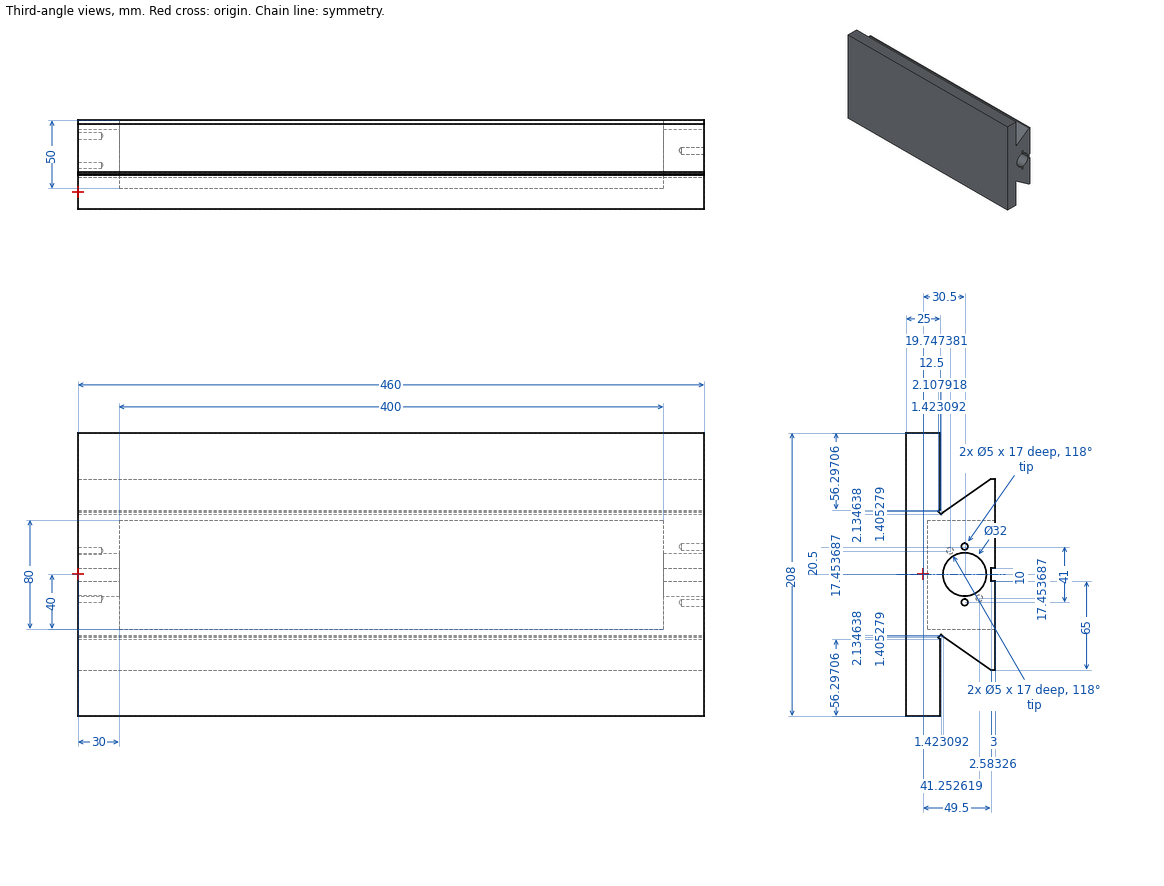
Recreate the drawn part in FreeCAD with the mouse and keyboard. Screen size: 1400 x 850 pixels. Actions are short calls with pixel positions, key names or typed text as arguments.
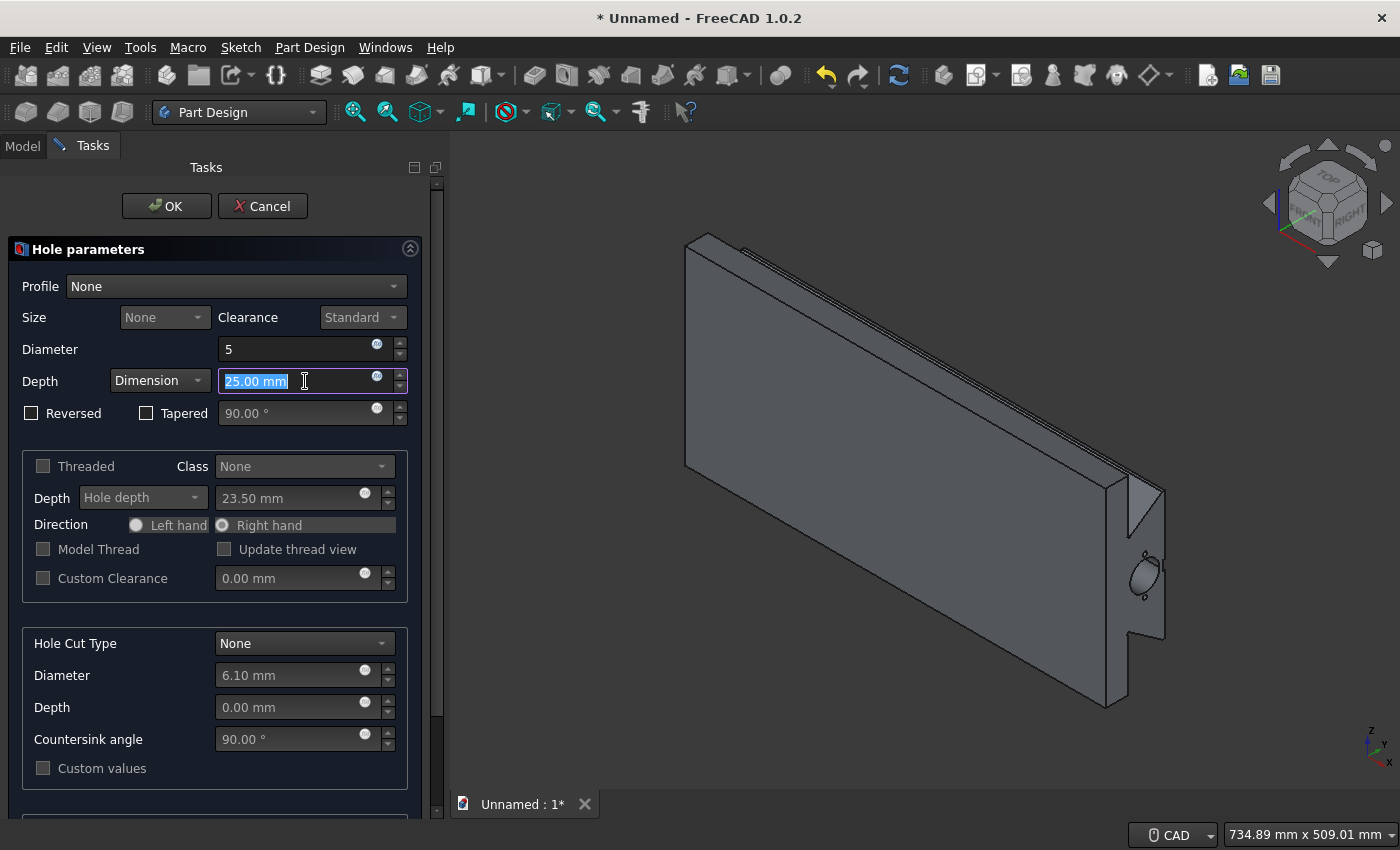
text(17)
key(Tab)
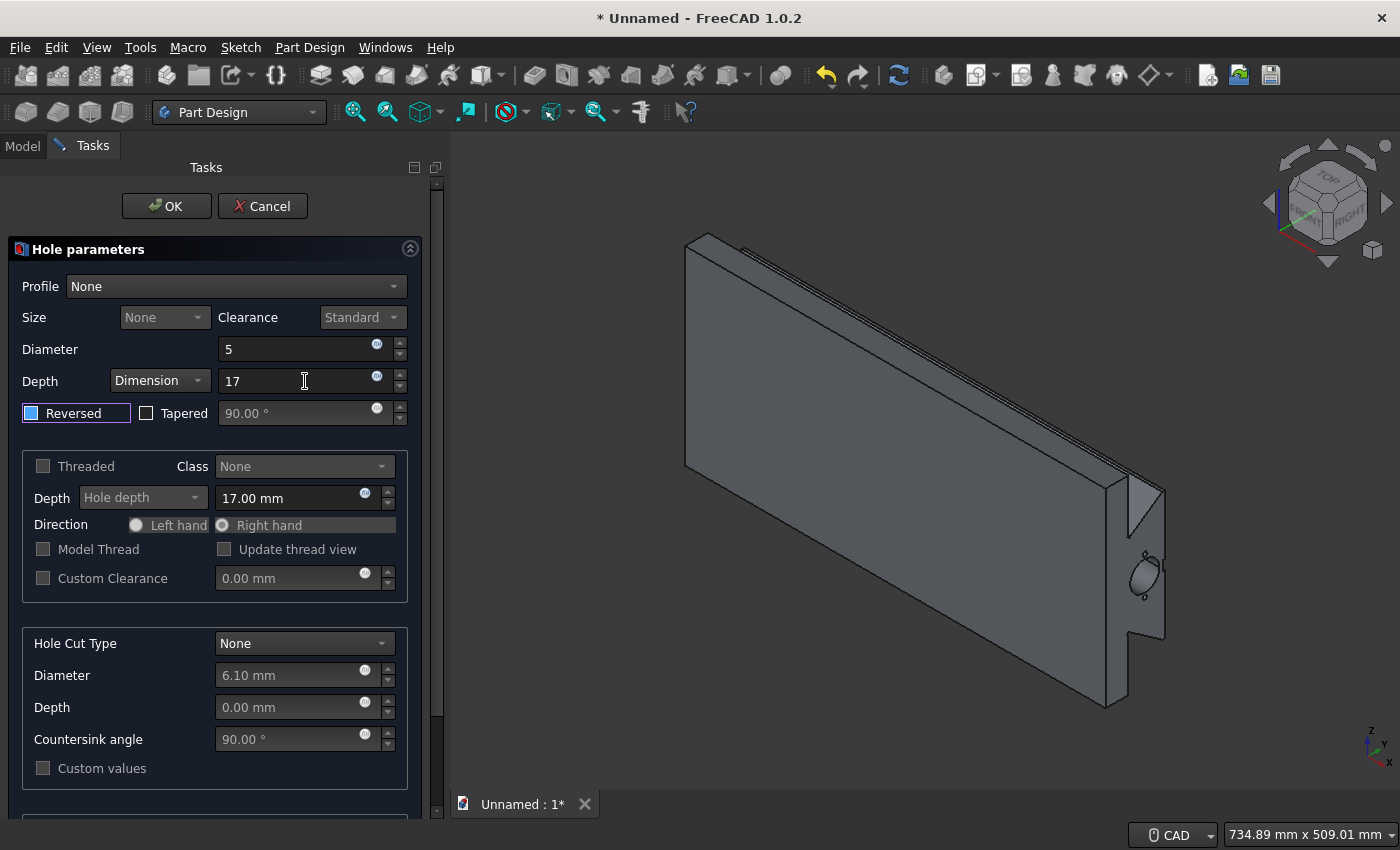
click(167, 206)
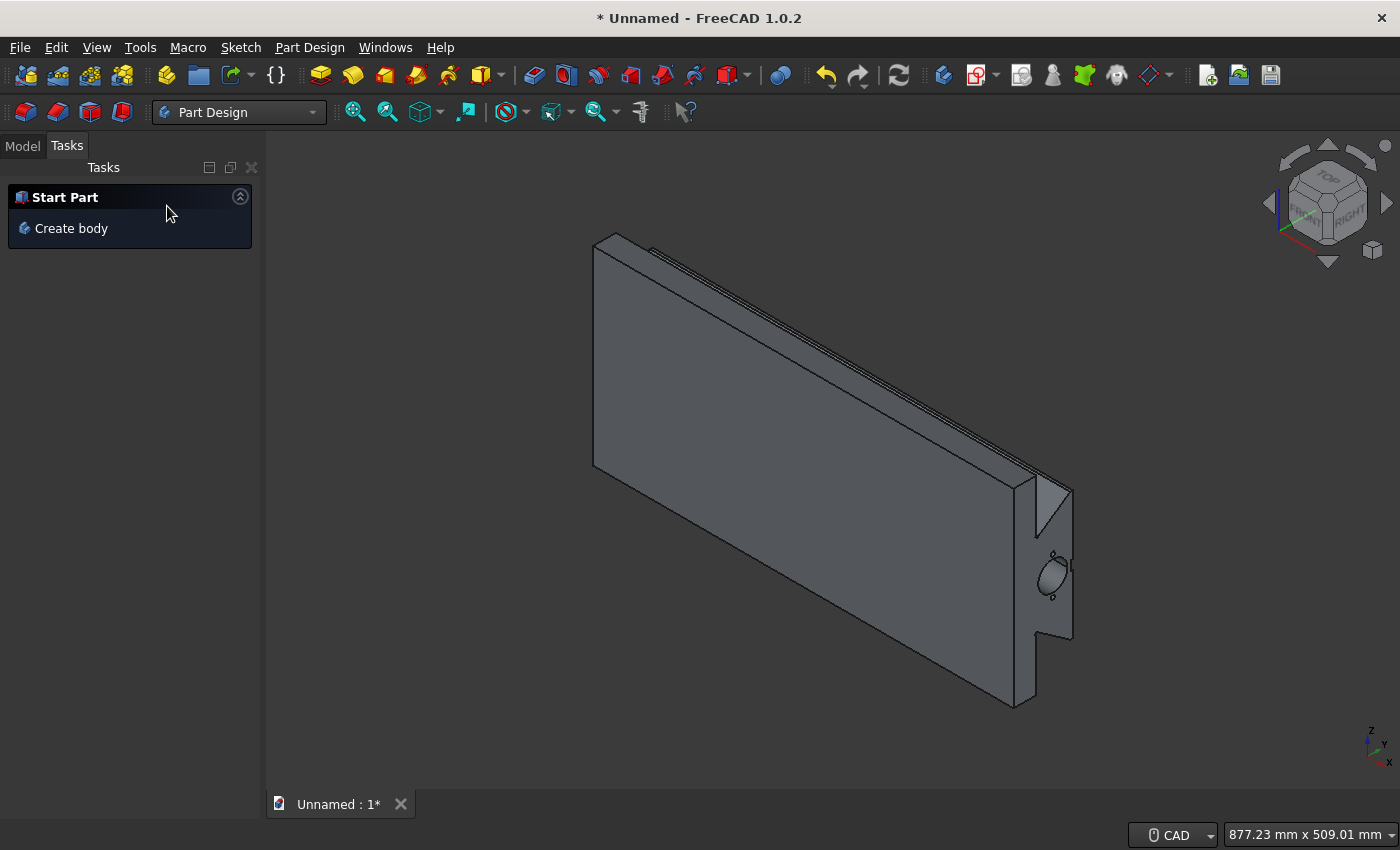
click(976, 76)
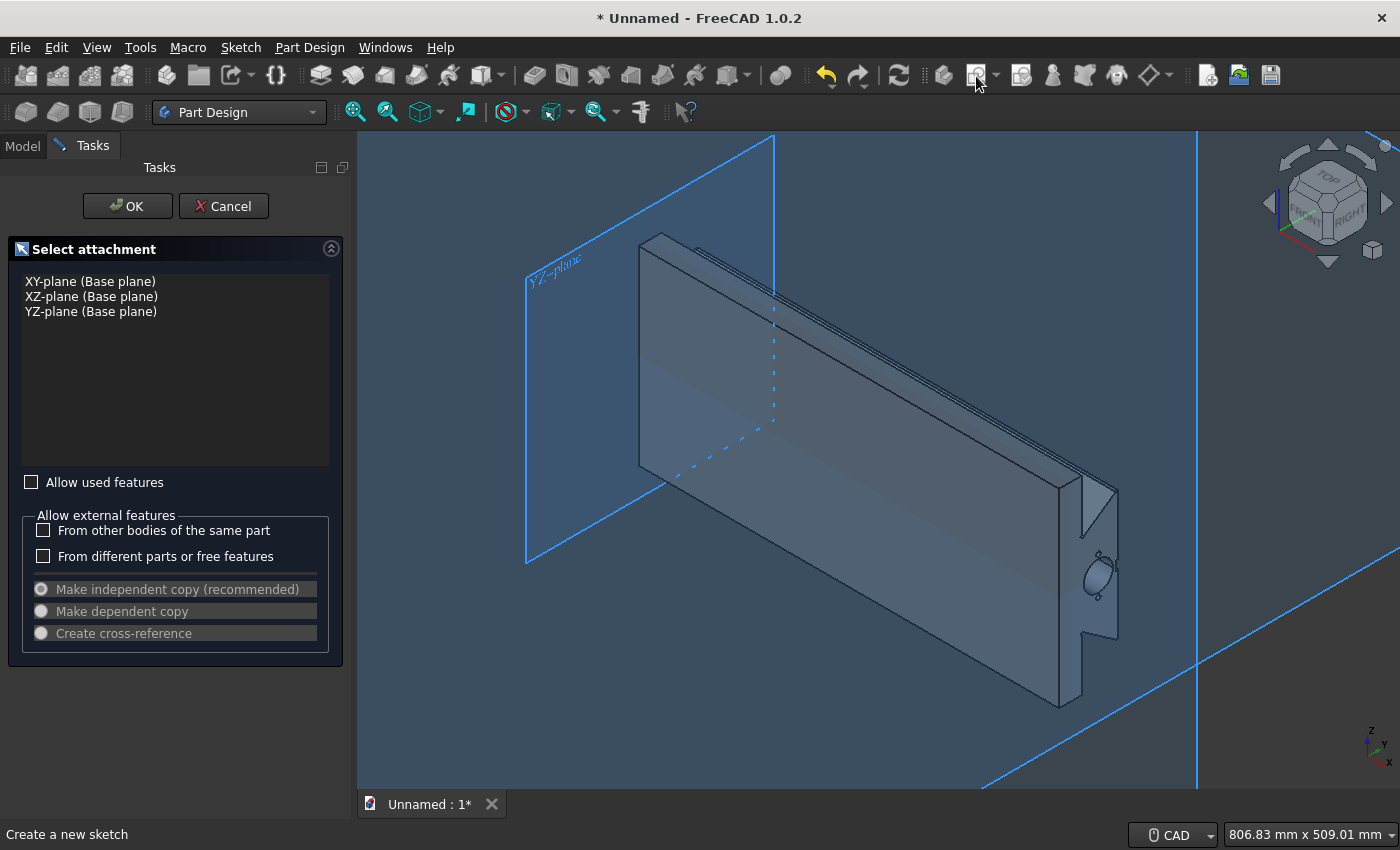
click(82, 312)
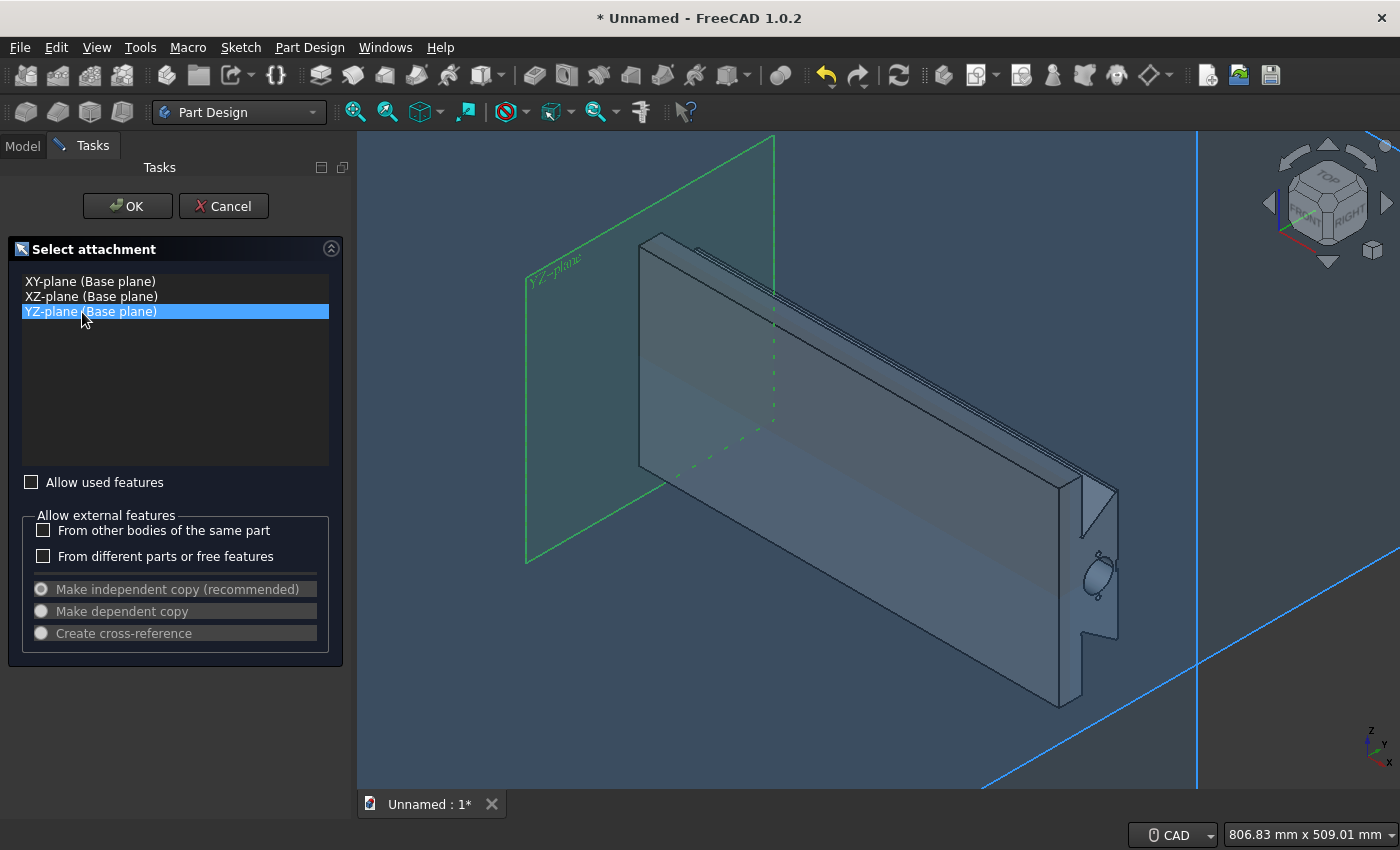
click(128, 206)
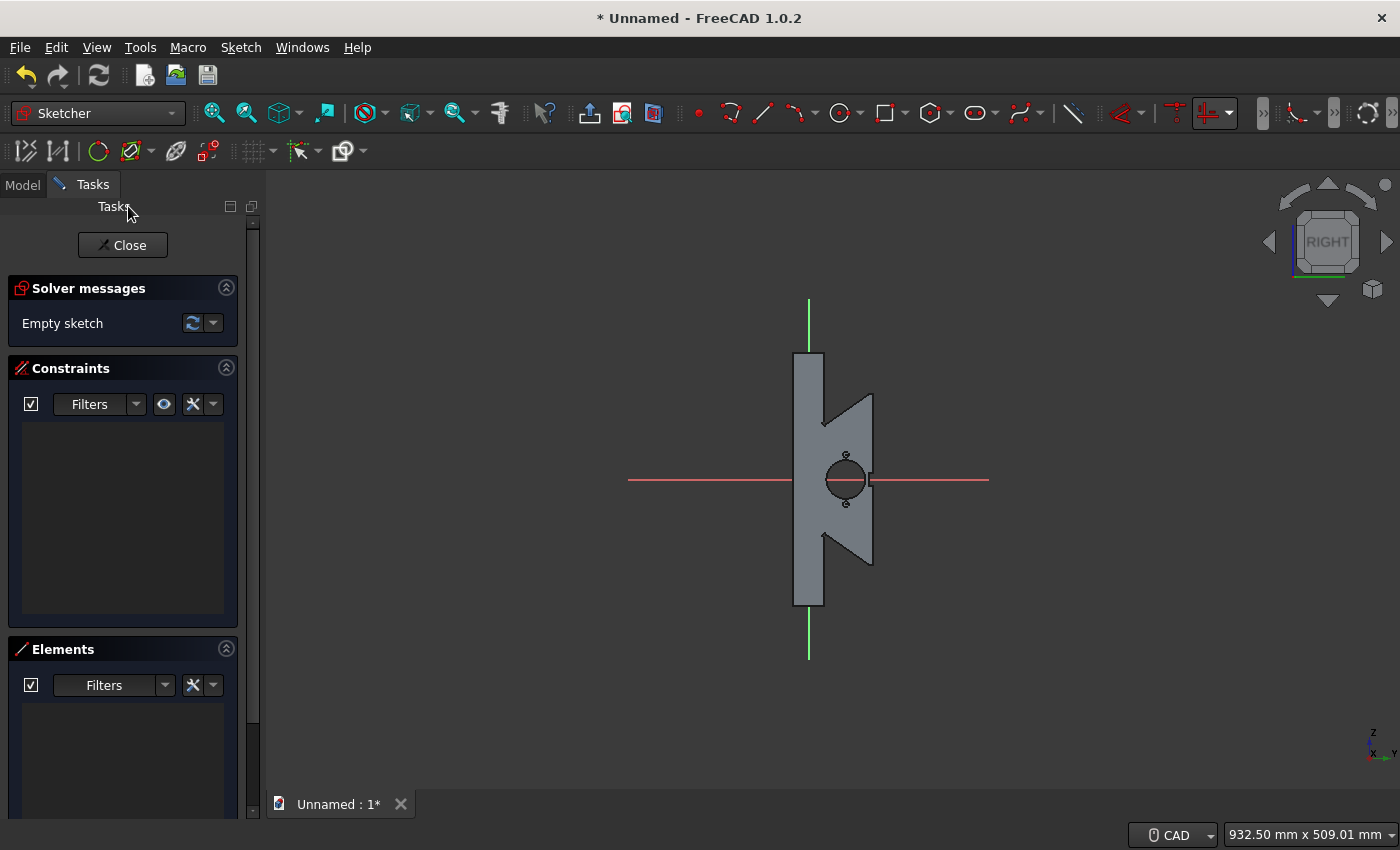
click(654, 114)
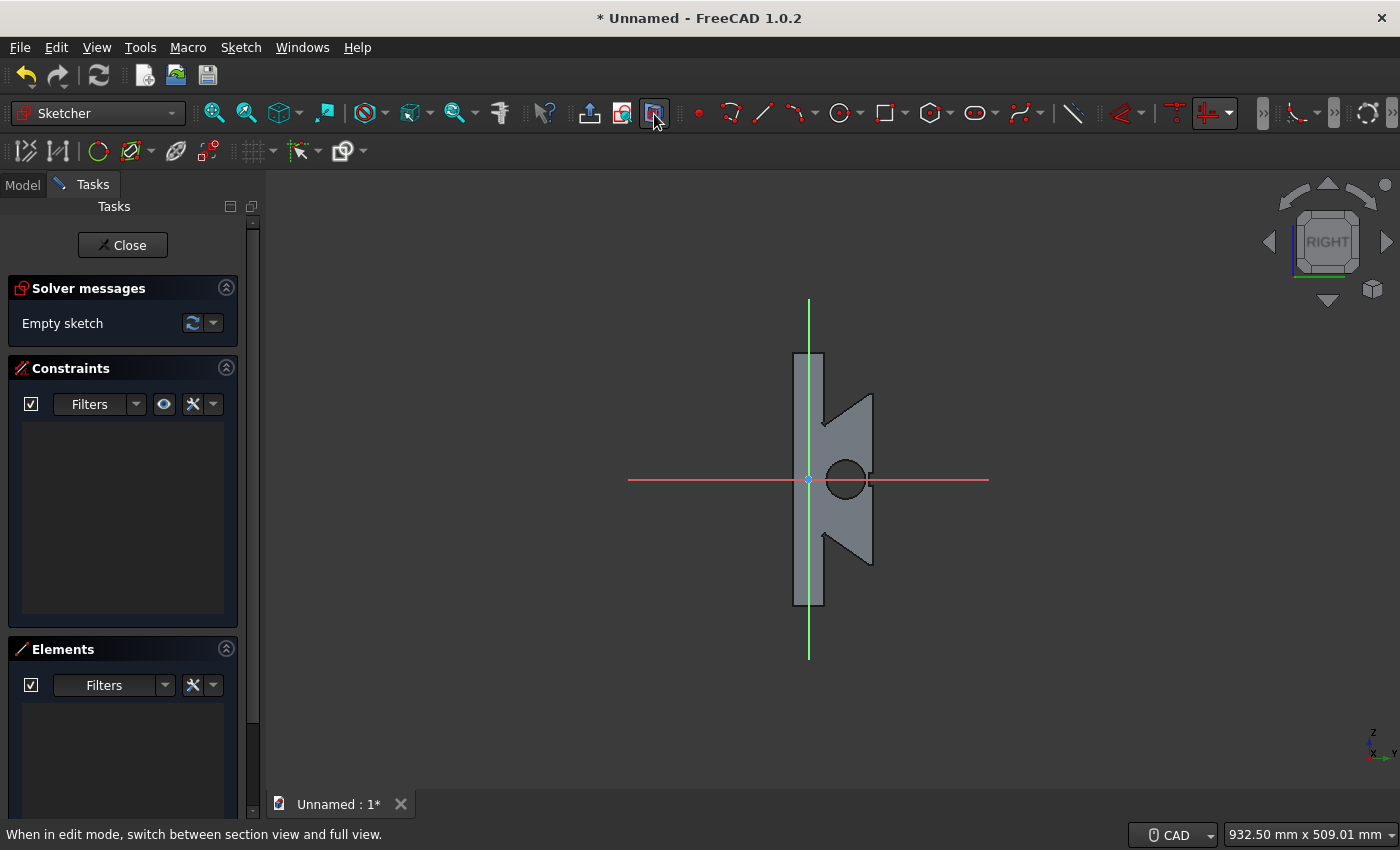
scroll(844, 480, up, 11)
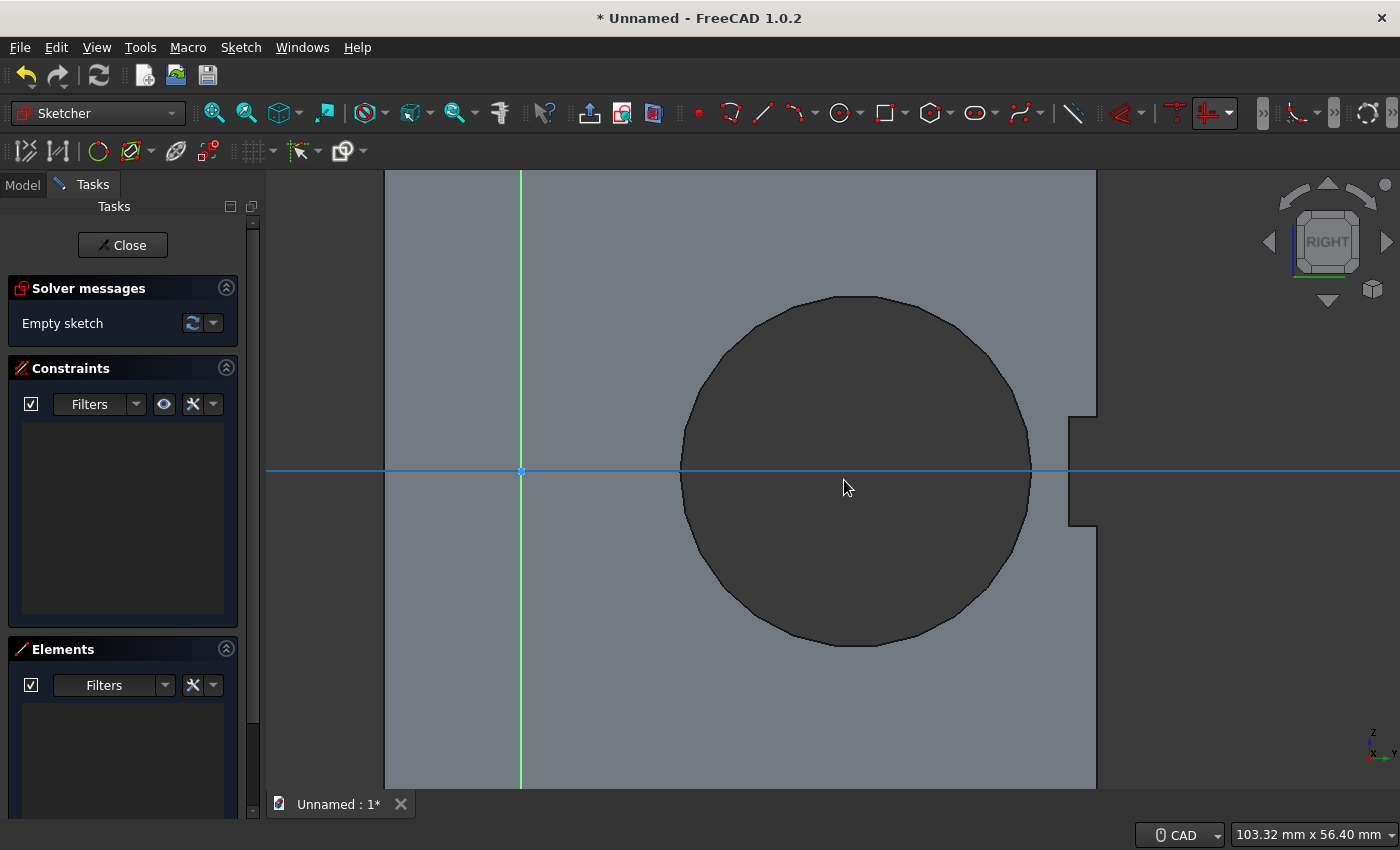
click(840, 114)